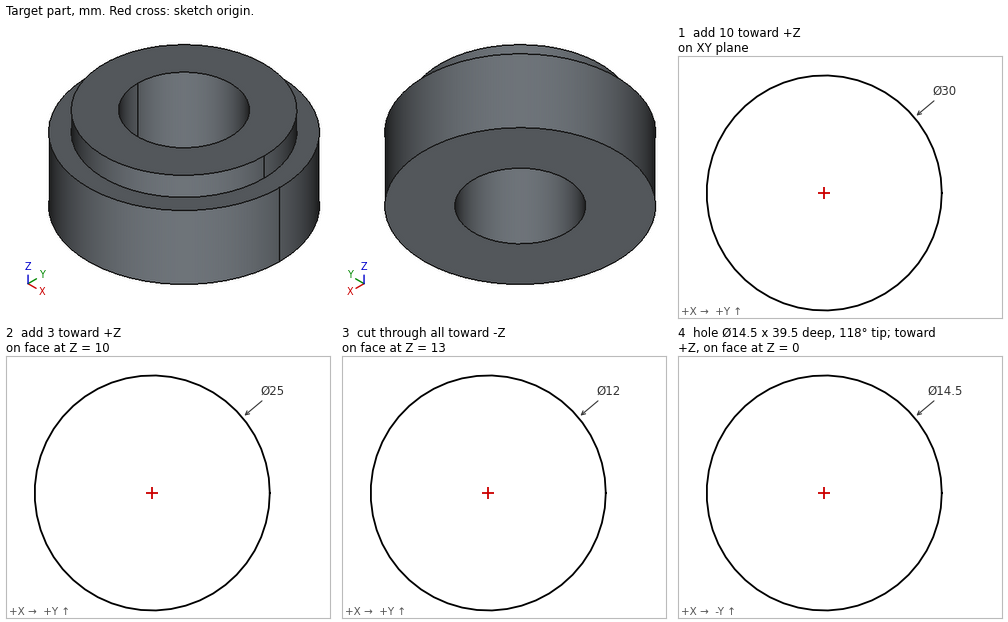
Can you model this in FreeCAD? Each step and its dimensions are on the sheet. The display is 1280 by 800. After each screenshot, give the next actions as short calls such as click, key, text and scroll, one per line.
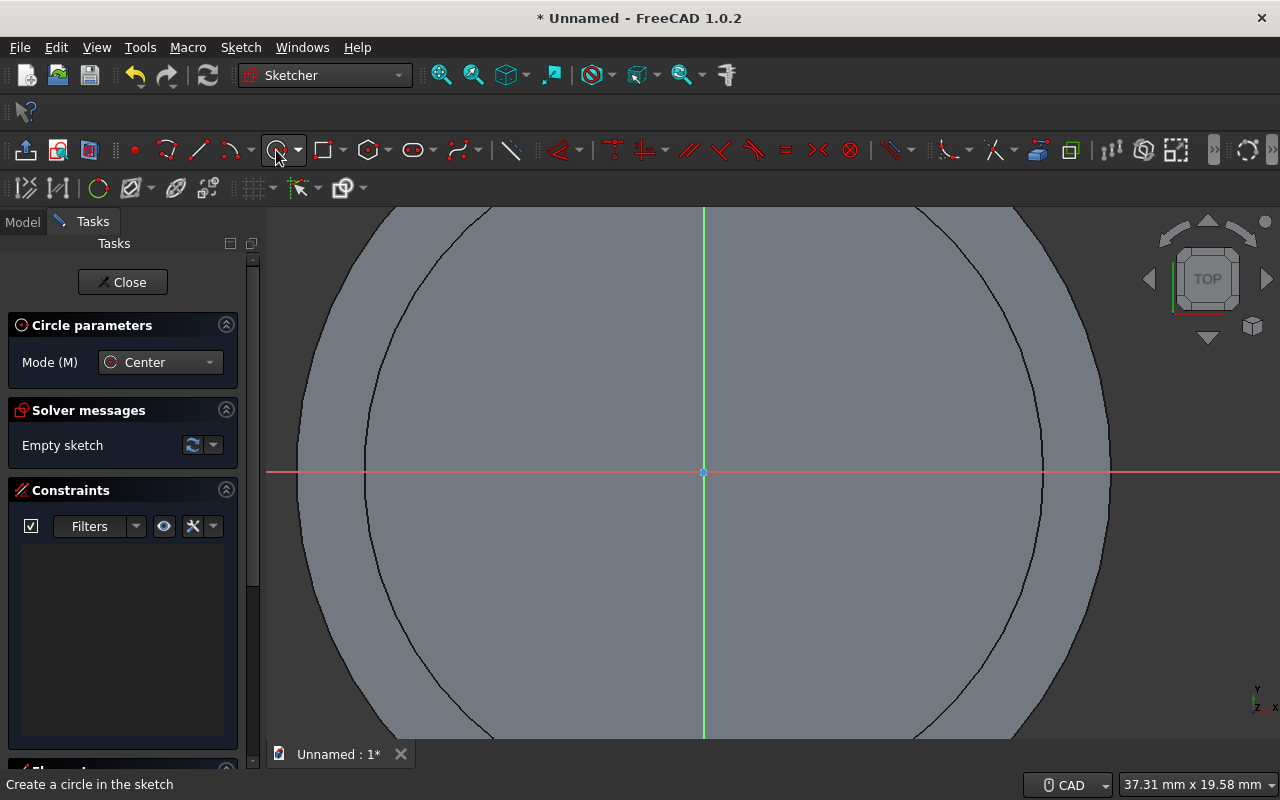
click(704, 472)
click(819, 357)
key(Escape)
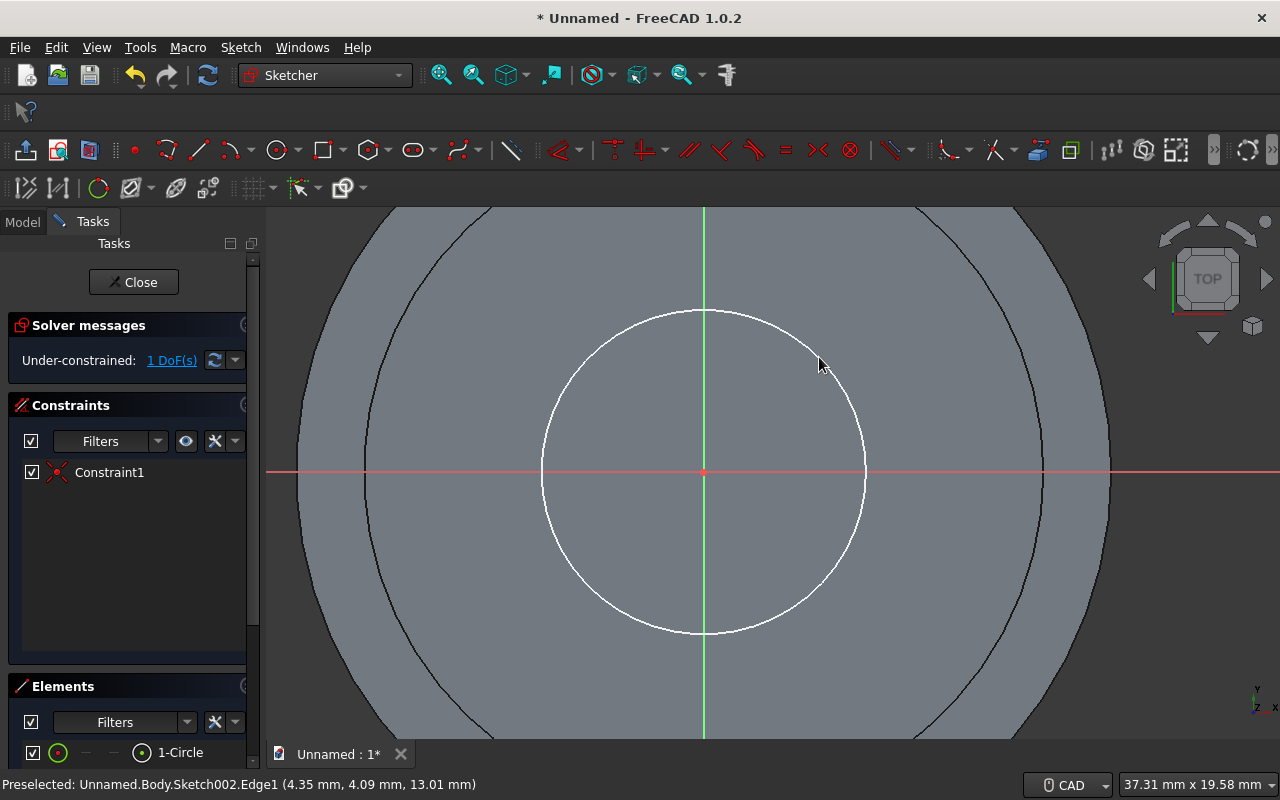
click(558, 150)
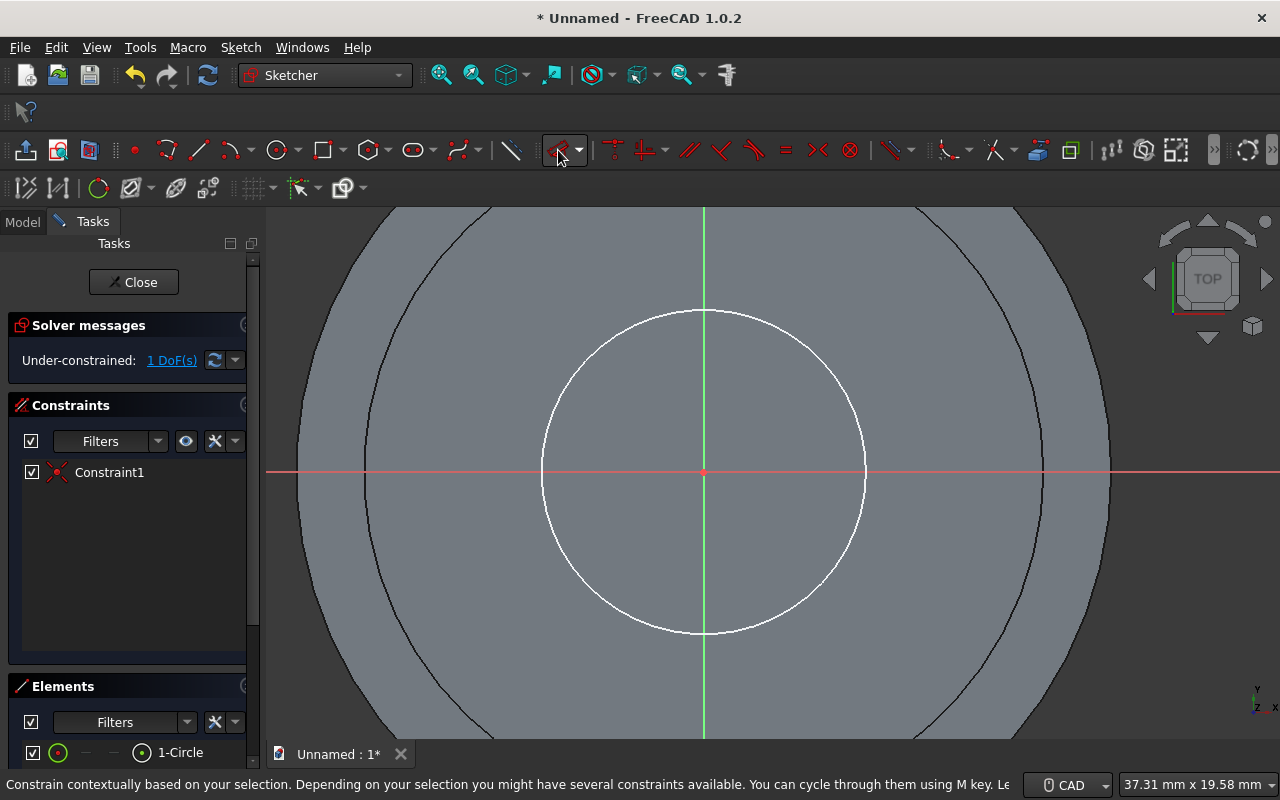
click(818, 357)
click(841, 334)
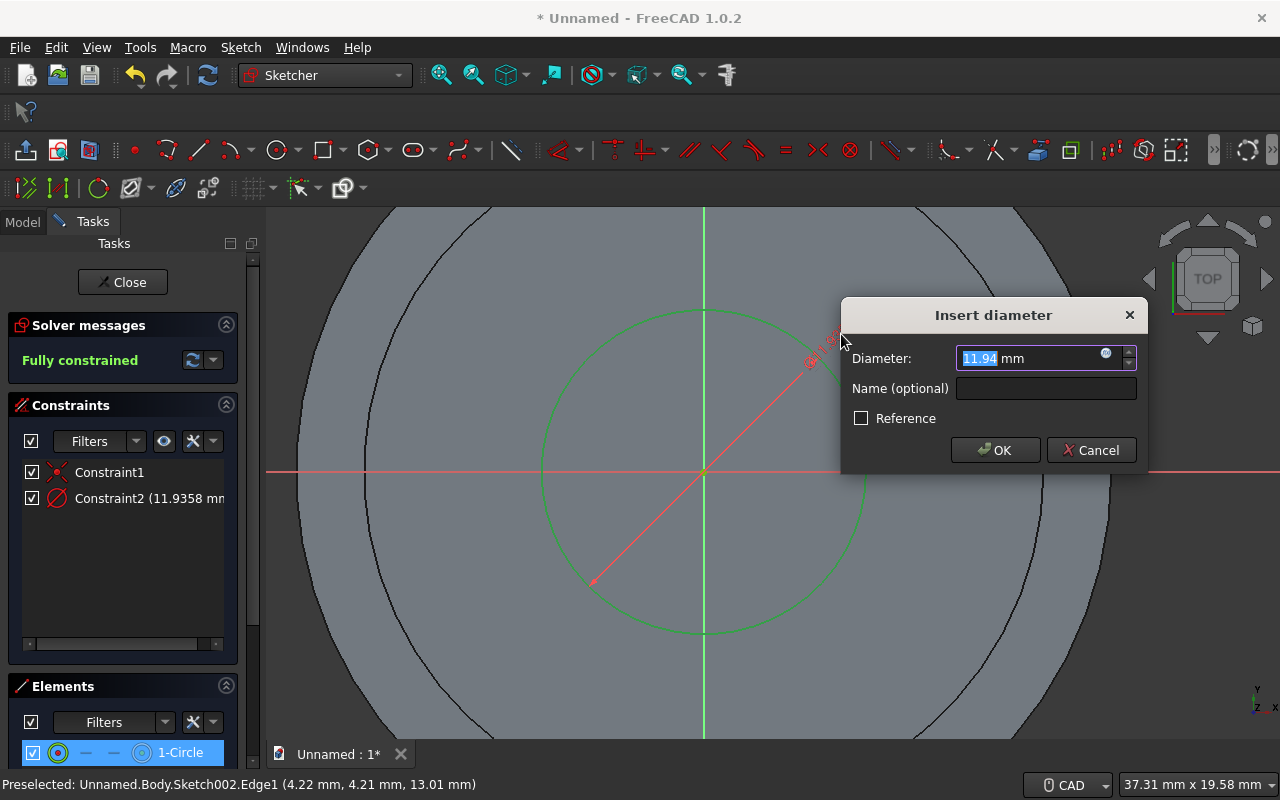
text(12)
key(Return)
key(Escape)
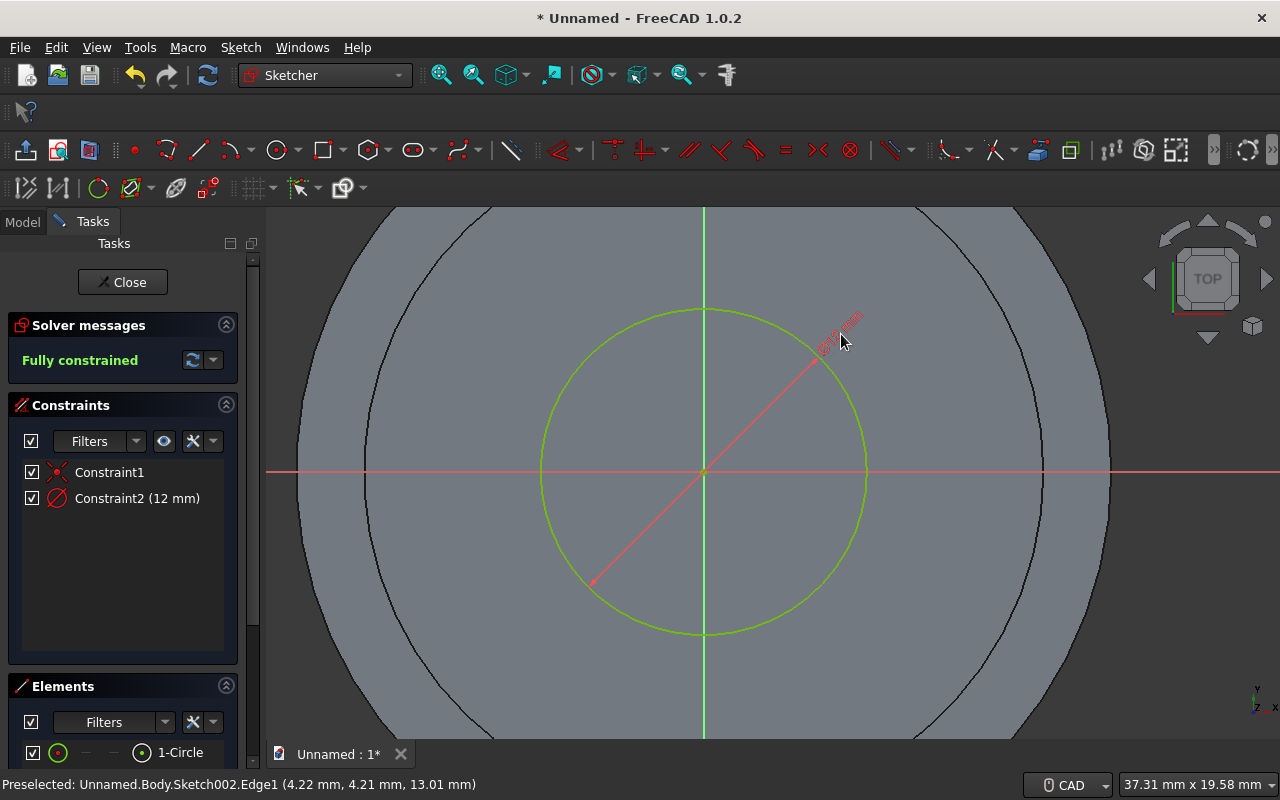
click(123, 282)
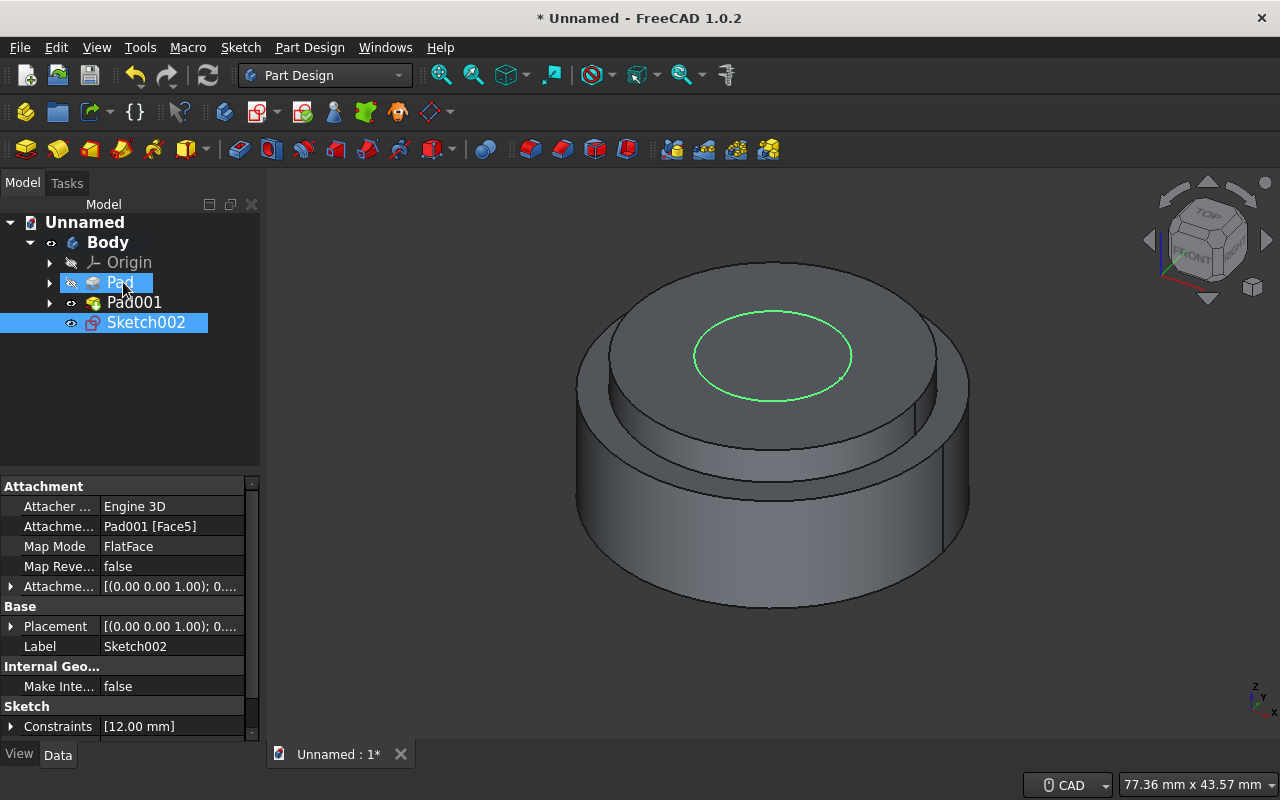
click(240, 150)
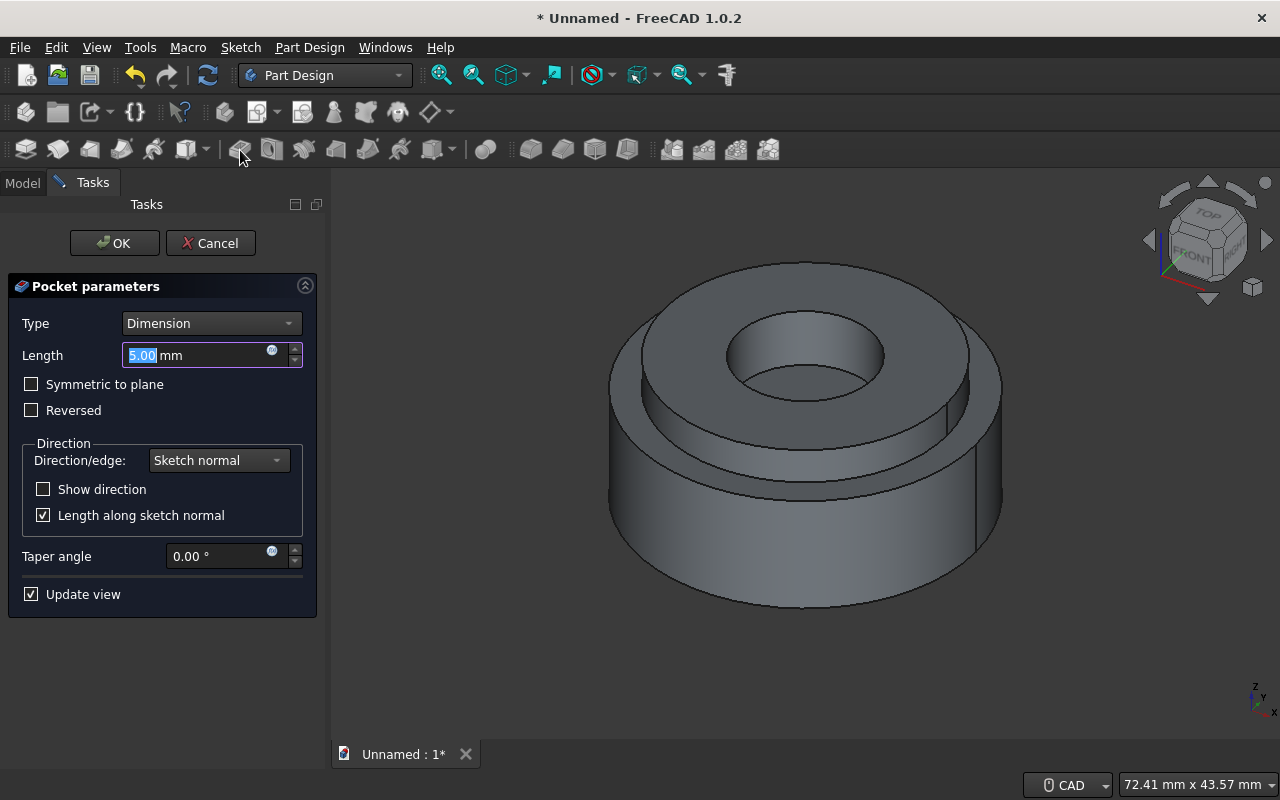
click(212, 324)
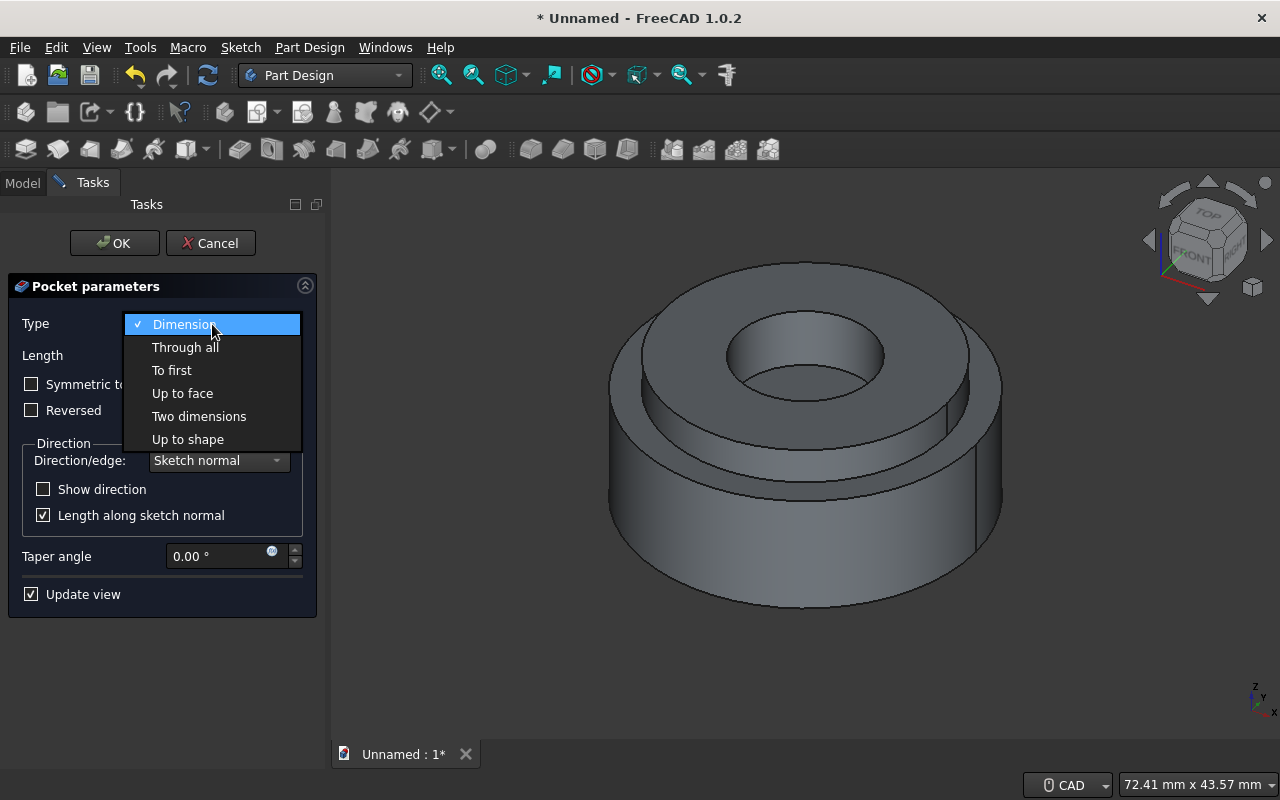
click(212, 348)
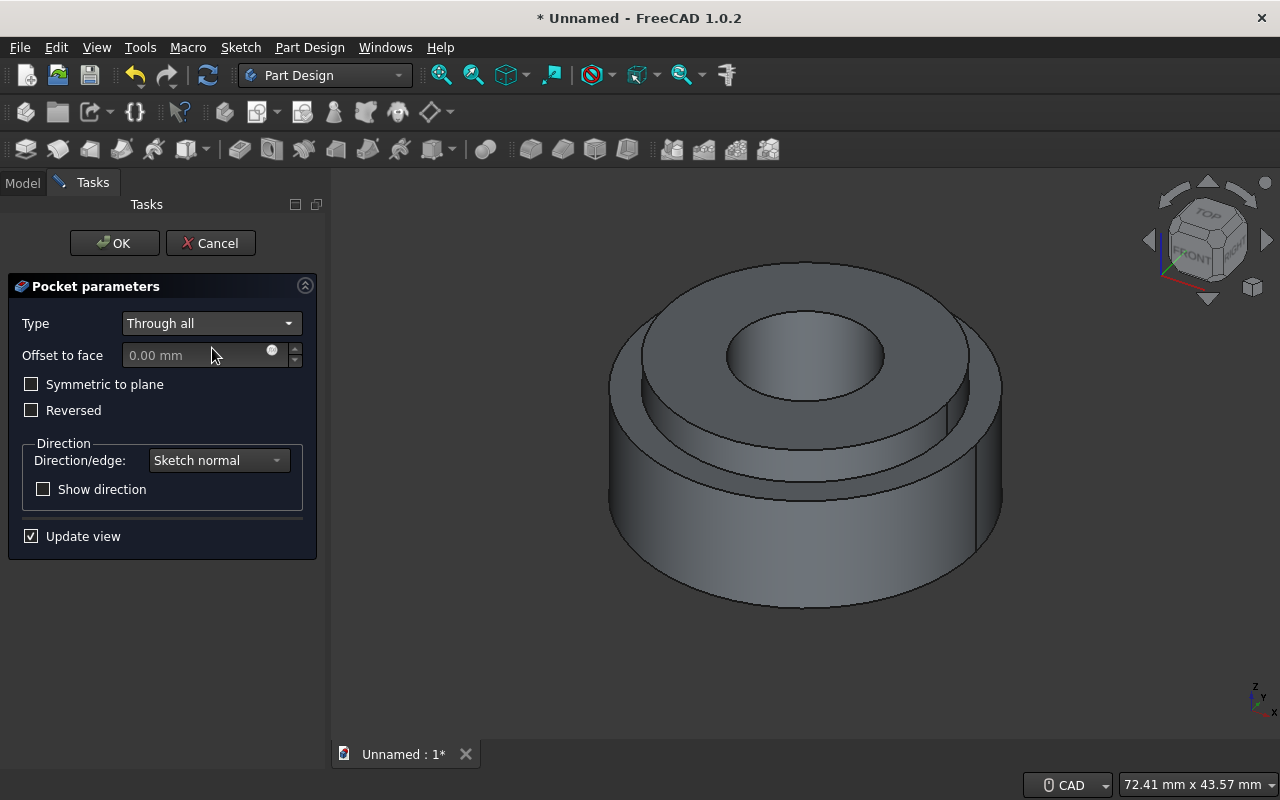
click(115, 243)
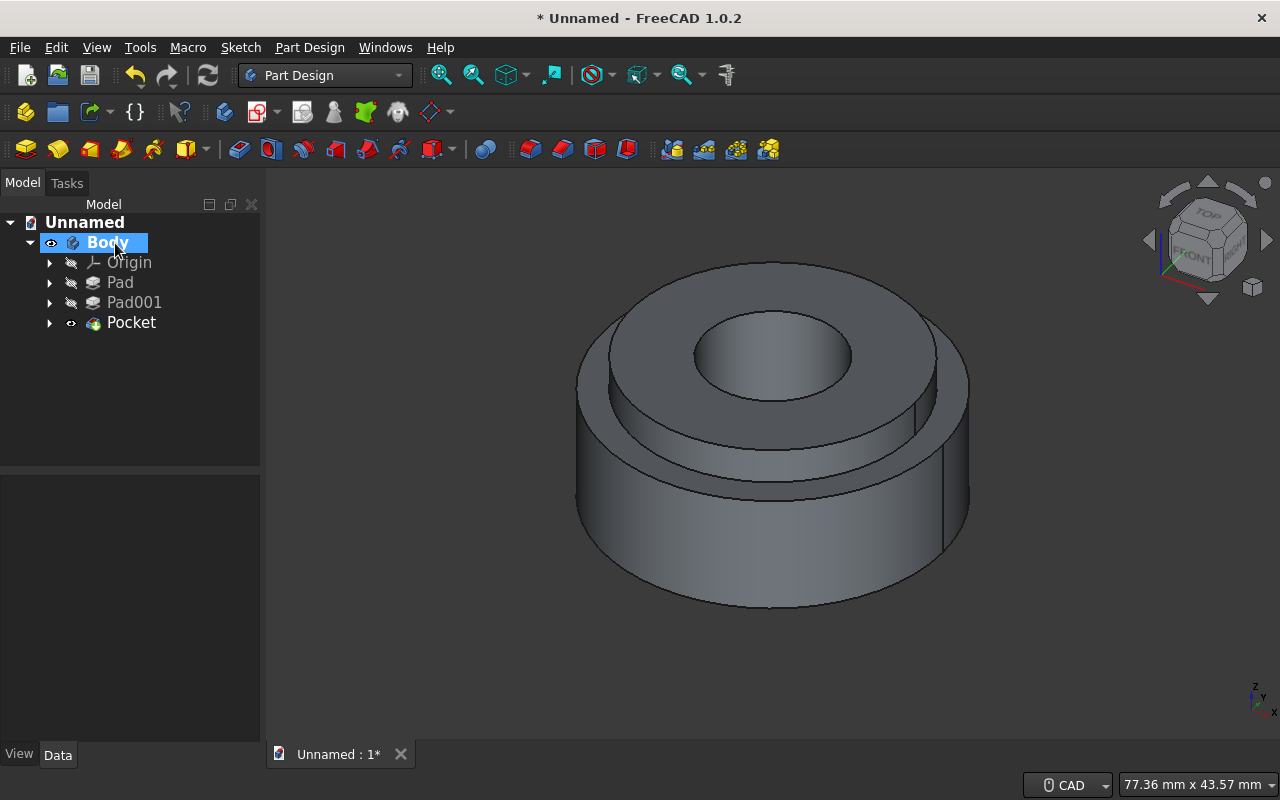
key(5)